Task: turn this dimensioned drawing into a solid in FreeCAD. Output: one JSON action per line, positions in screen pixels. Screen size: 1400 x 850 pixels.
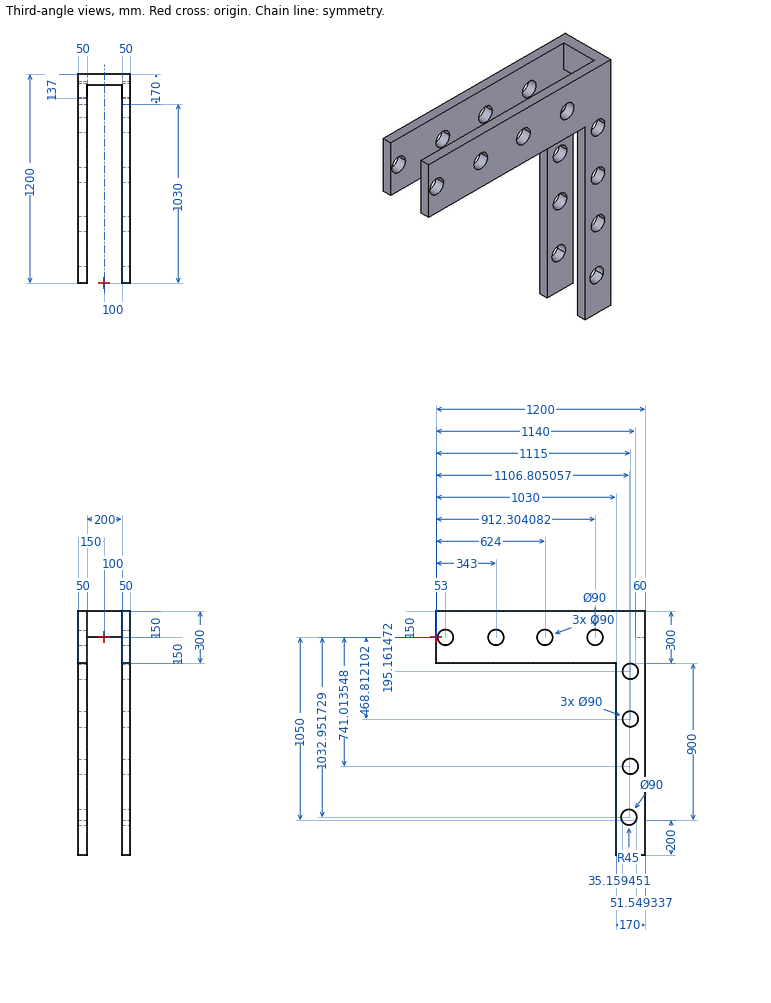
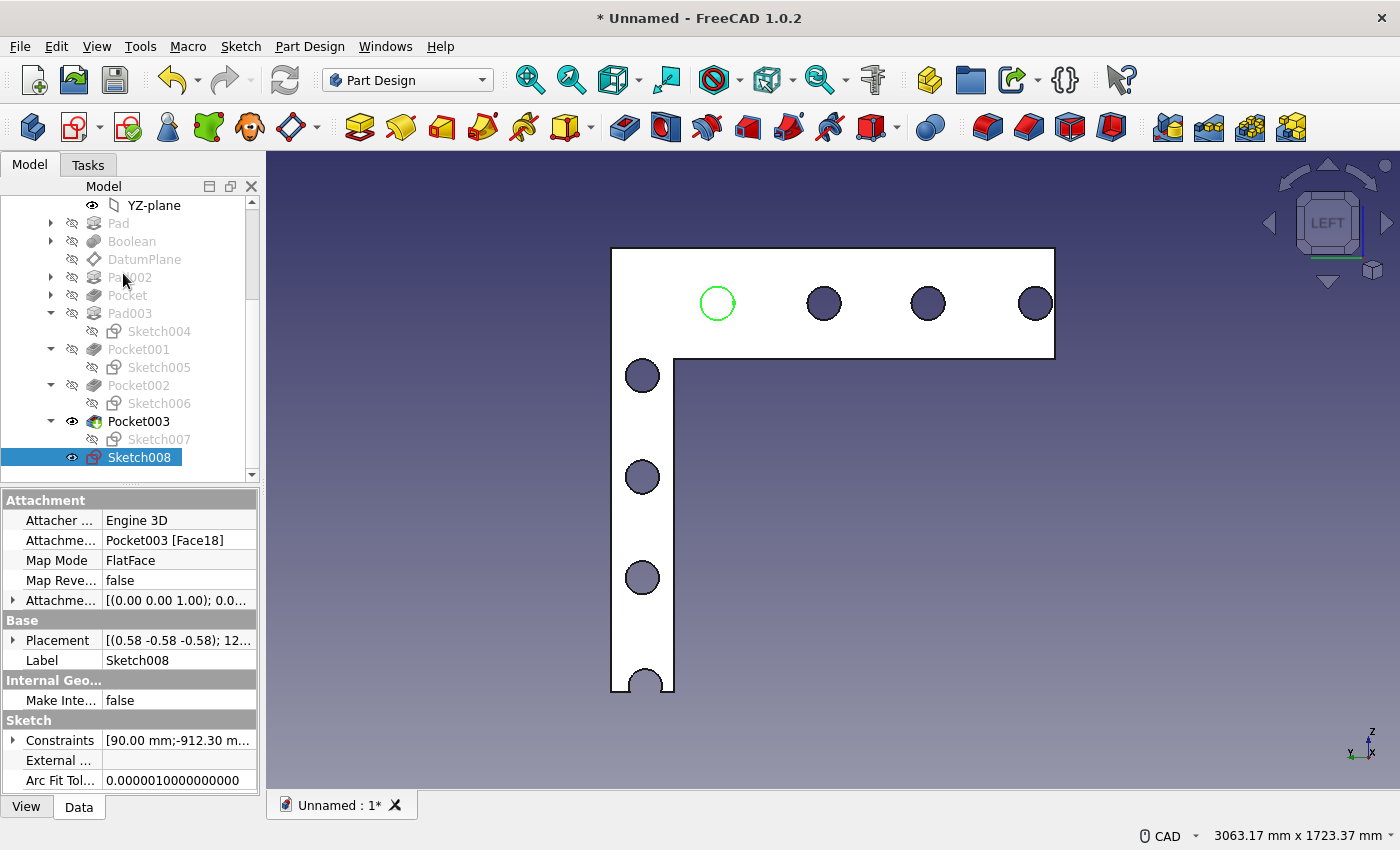
{"action": "left_click", "coordinate": [625, 128]}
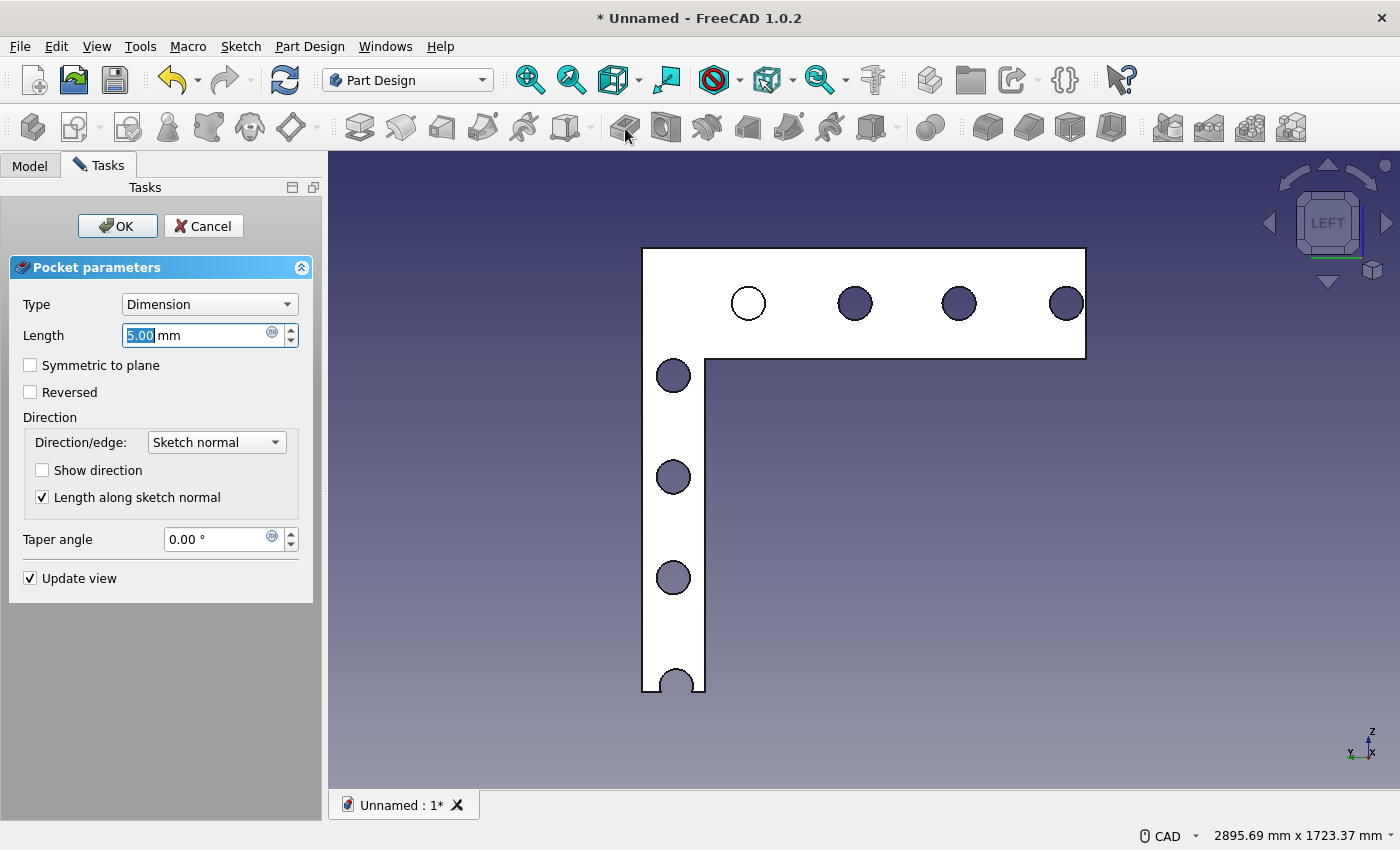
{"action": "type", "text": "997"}
{"action": "key", "text": "Tab"}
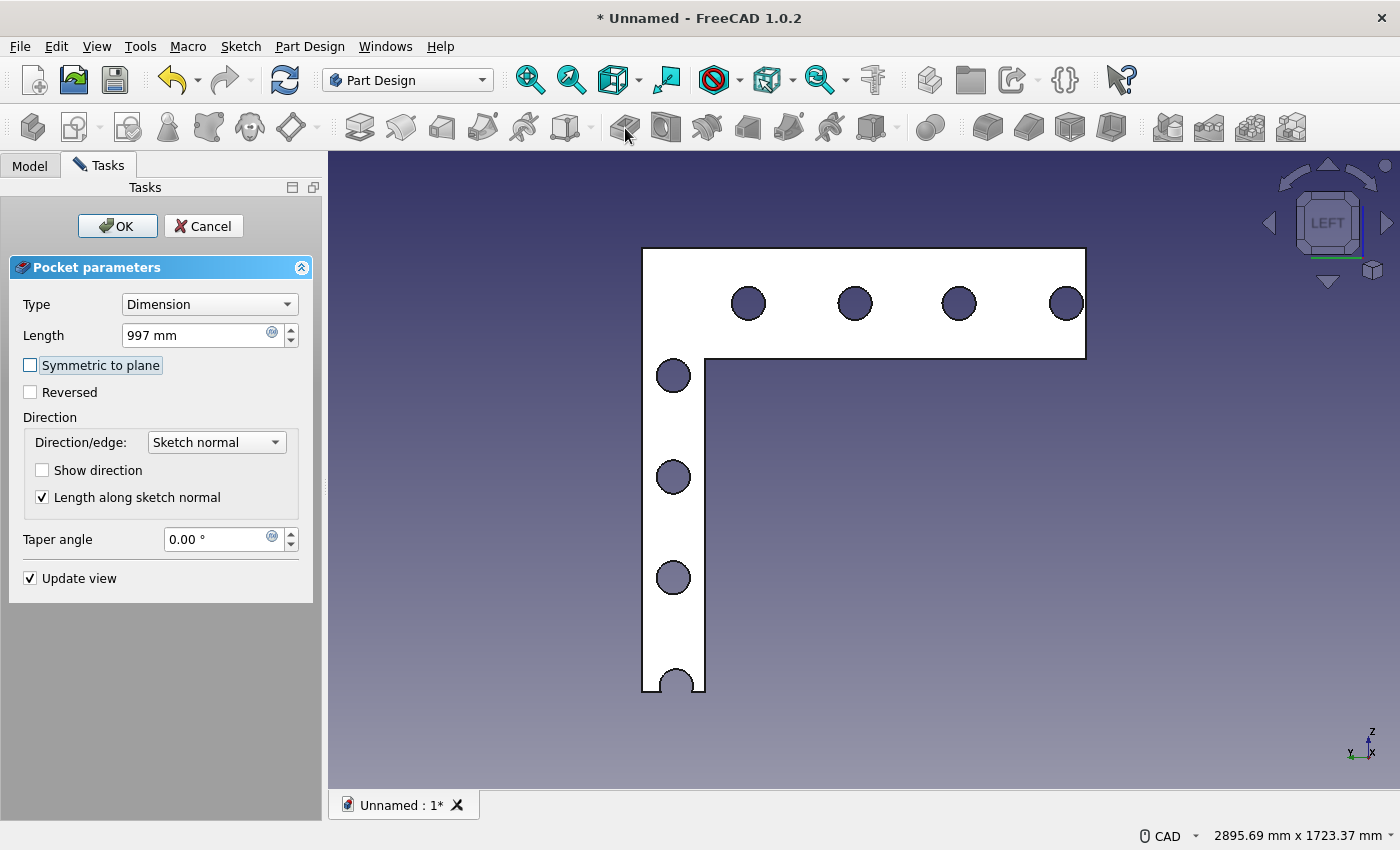
{"action": "left_click", "coordinate": [118, 226]}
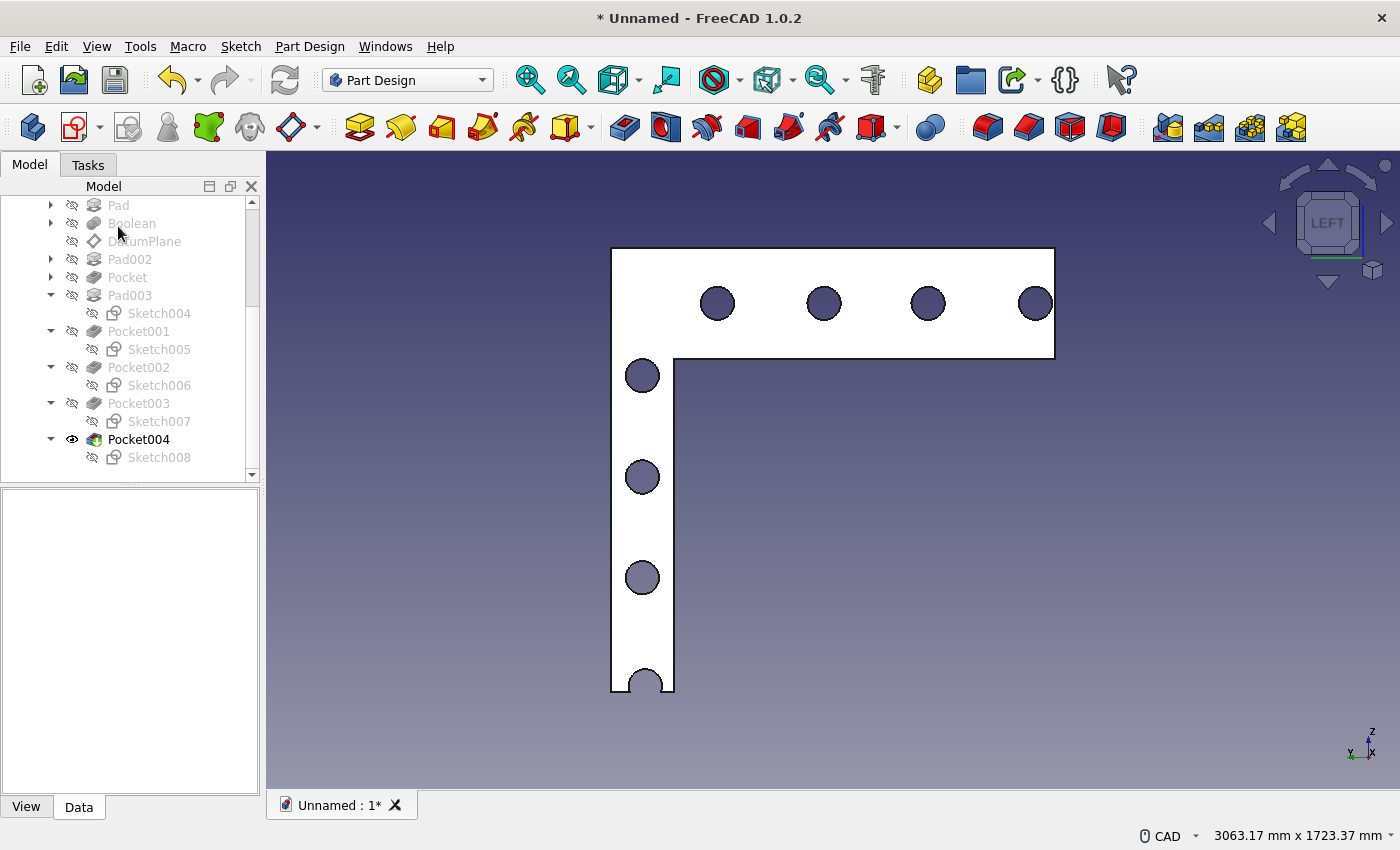
{"action": "scroll", "coordinate": [141, 327], "scroll_direction": "down", "scroll_amount": 3}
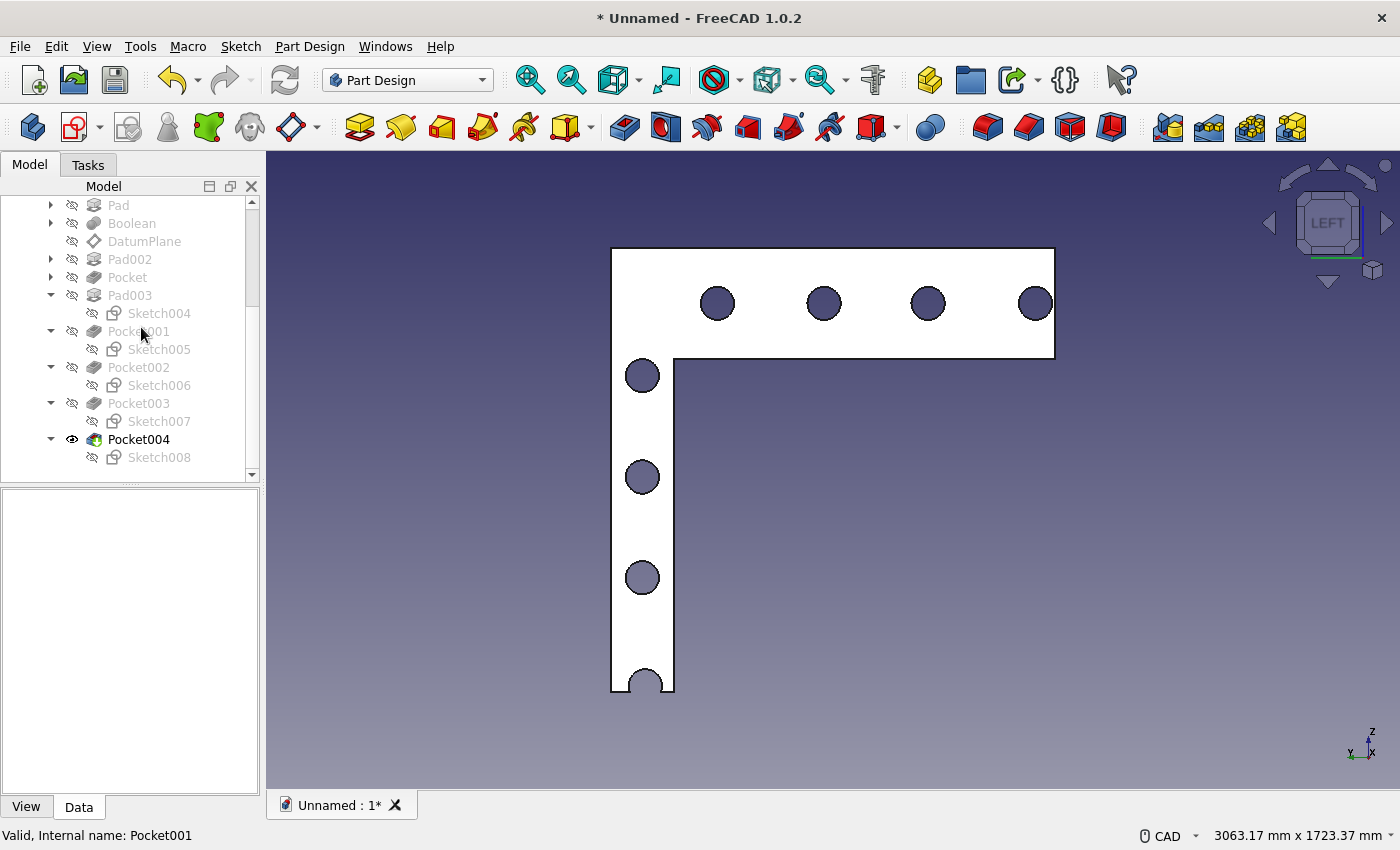
{"action": "scroll", "coordinate": [141, 327], "scroll_direction": "up", "scroll_amount": 15}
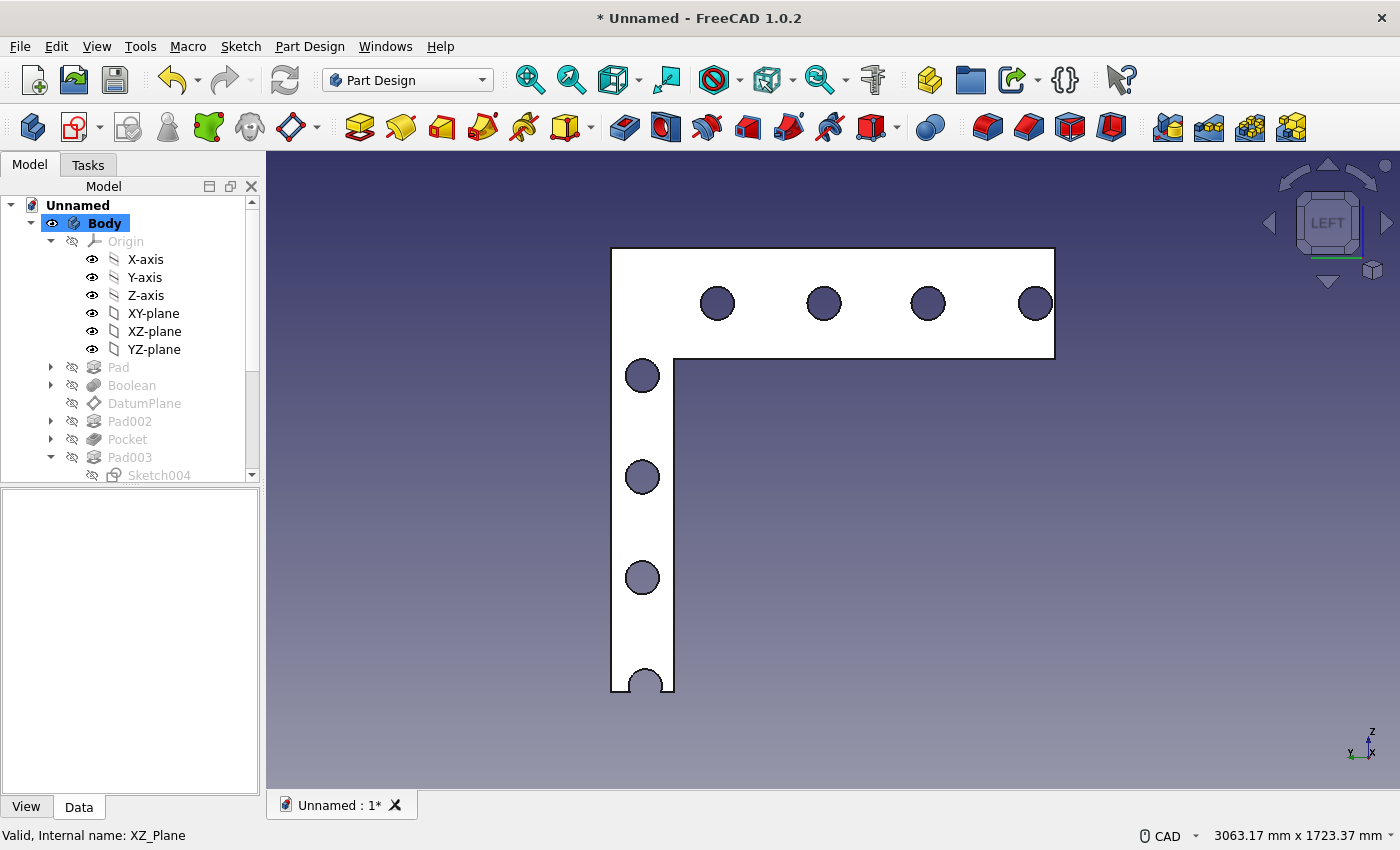
{"action": "left_click", "coordinate": [137, 349]}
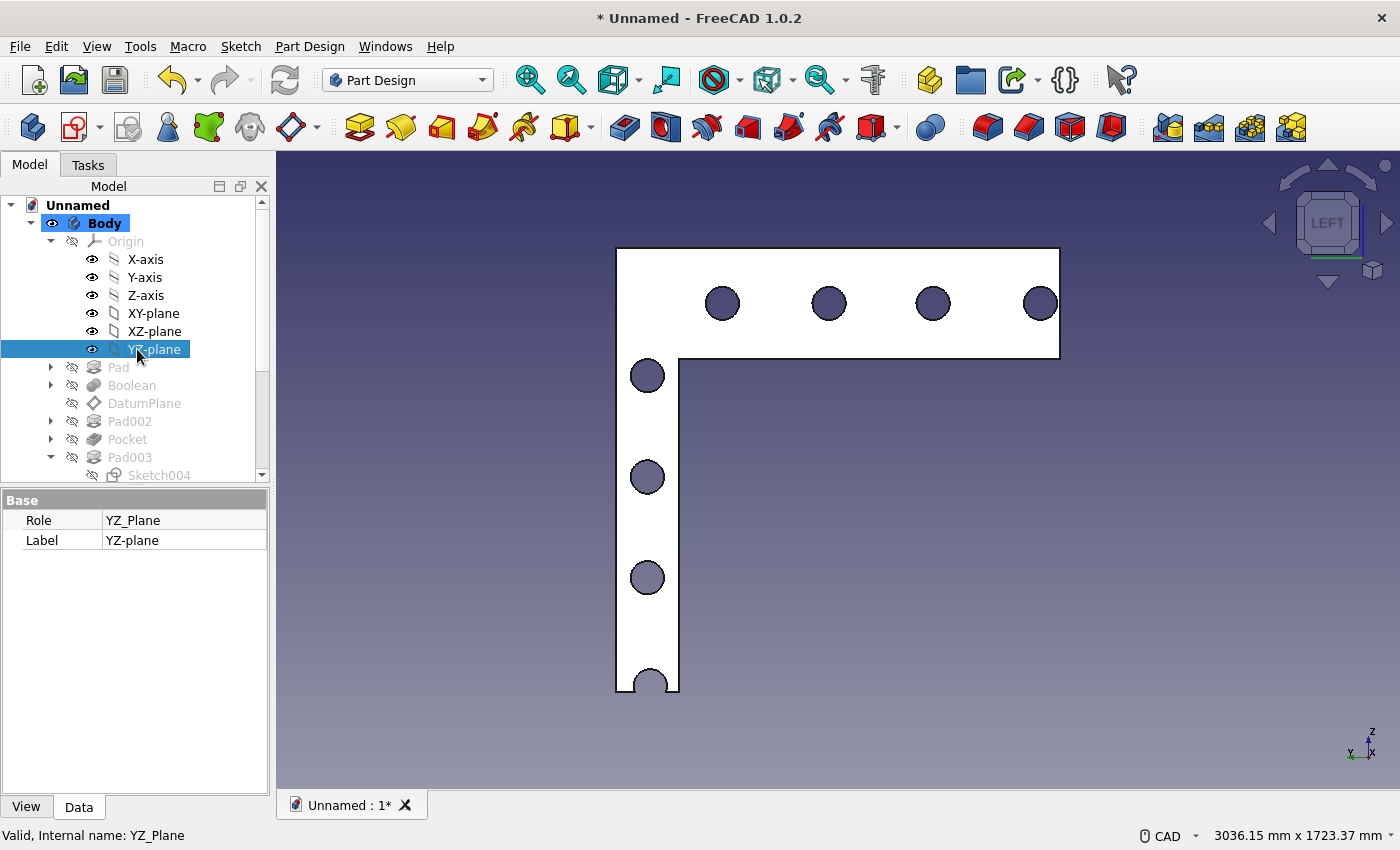
{"action": "left_click", "coordinate": [290, 128]}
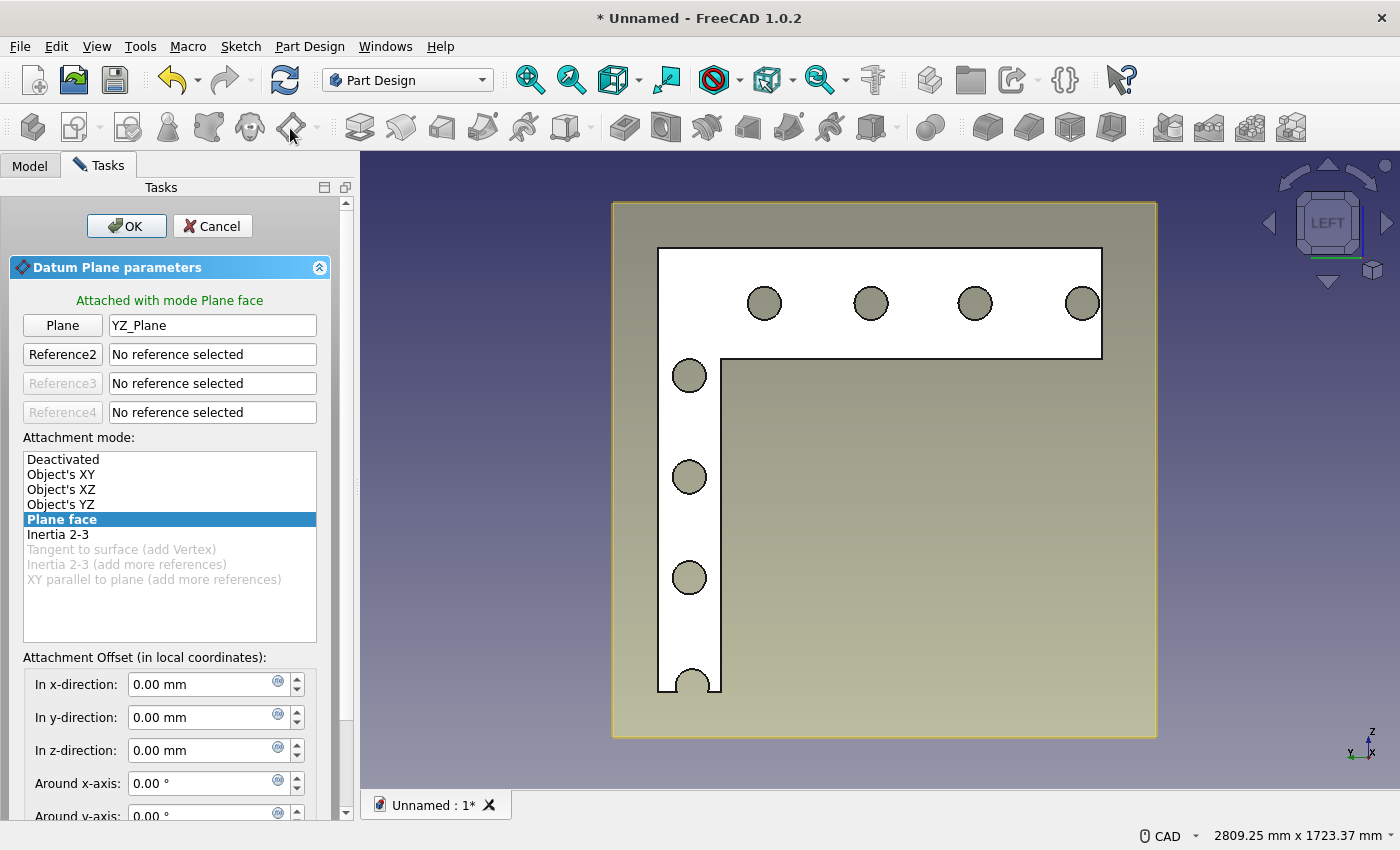
{"action": "triple_click", "coordinate": [210, 750]}